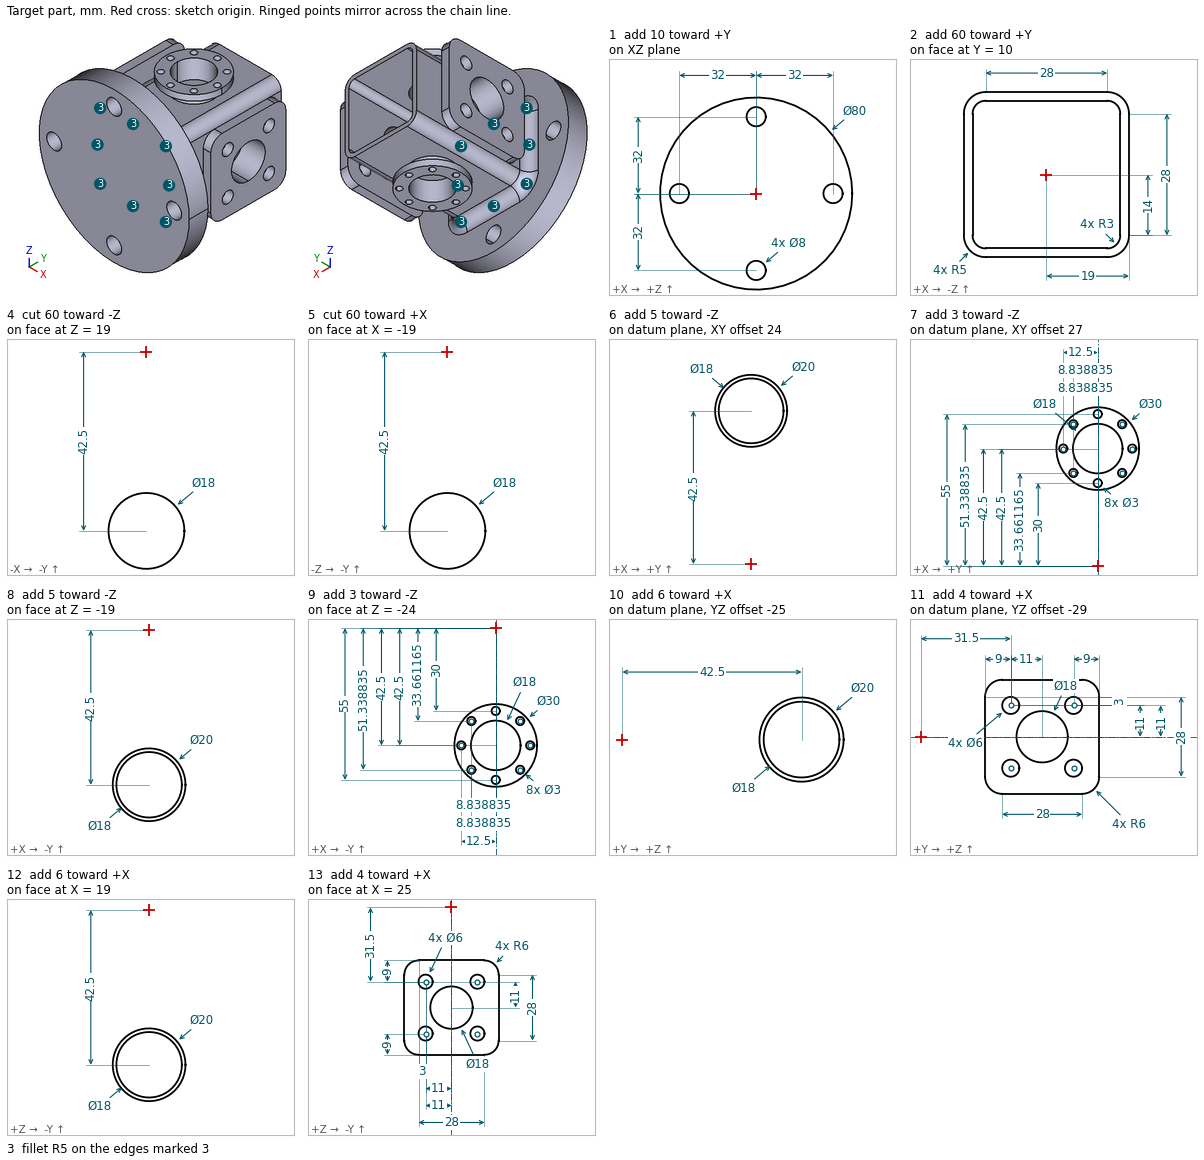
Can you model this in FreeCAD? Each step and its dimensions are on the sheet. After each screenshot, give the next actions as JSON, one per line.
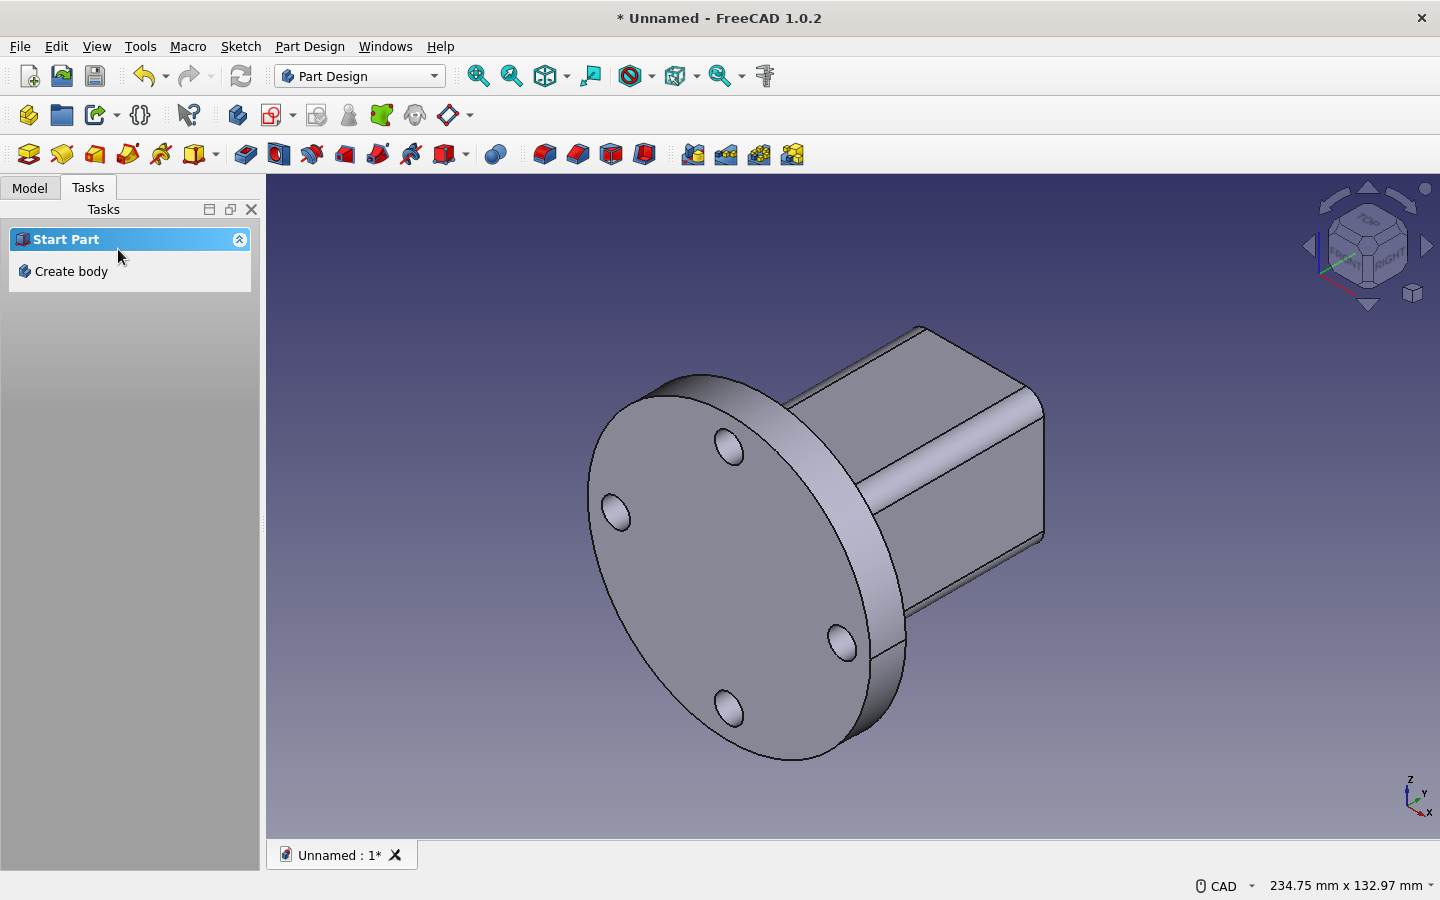
{"action": "key", "text": "2"}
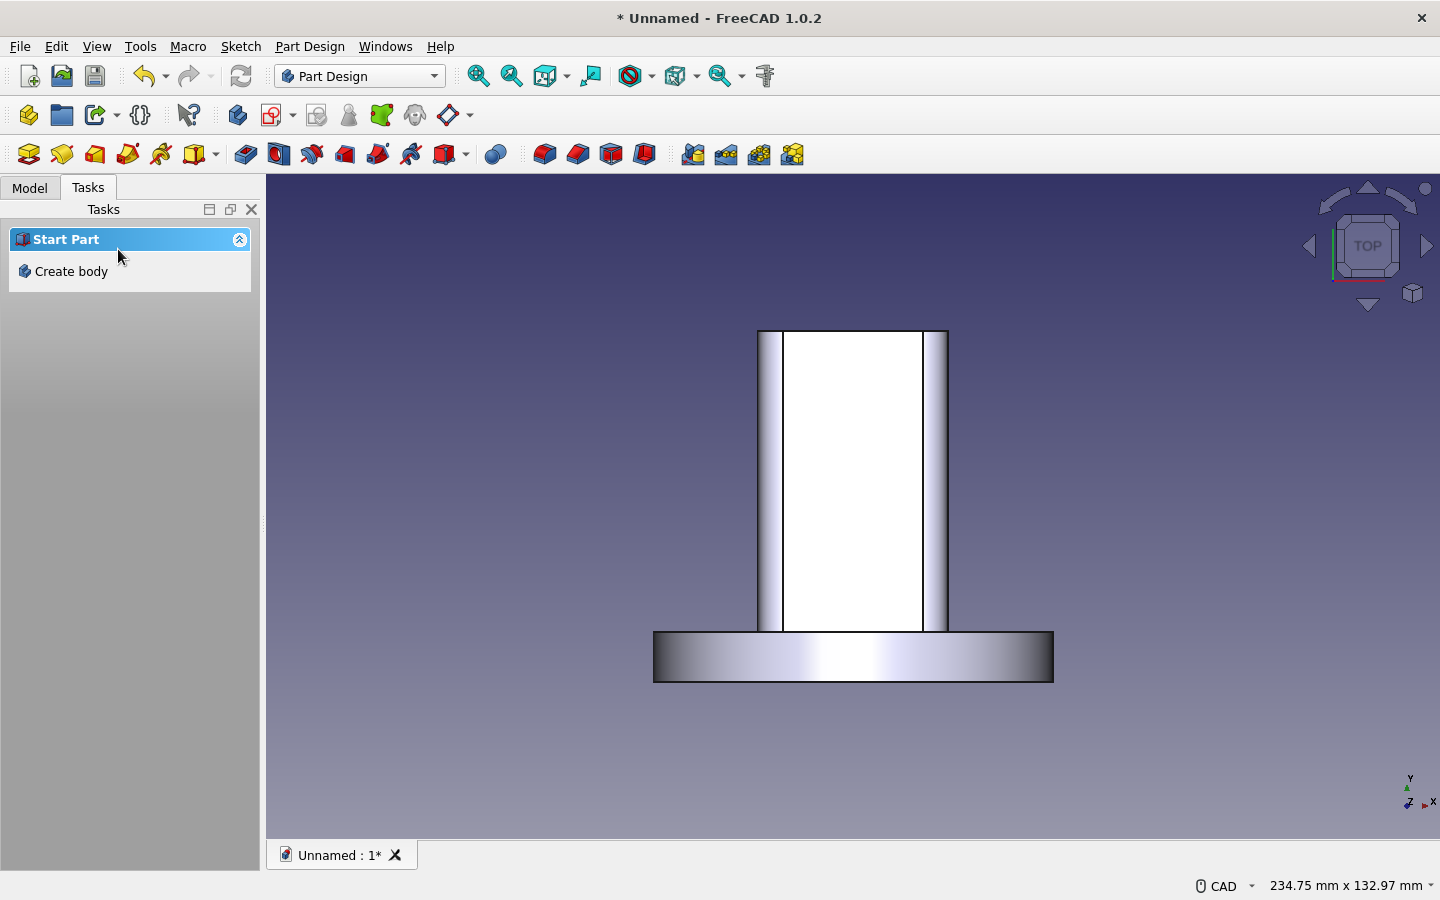
{"action": "key", "text": "1"}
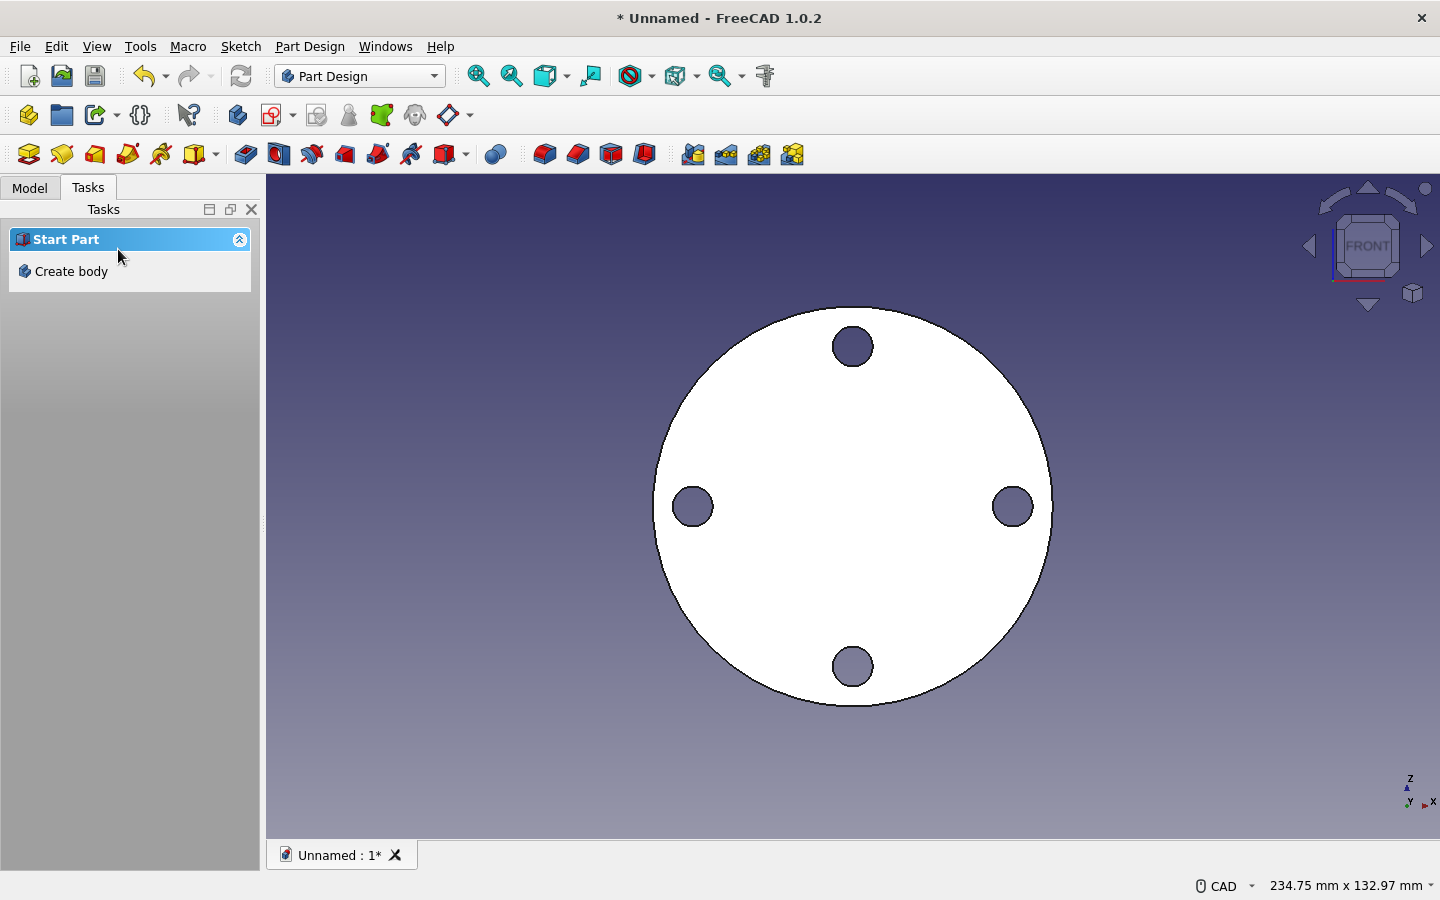
{"action": "key", "text": "3"}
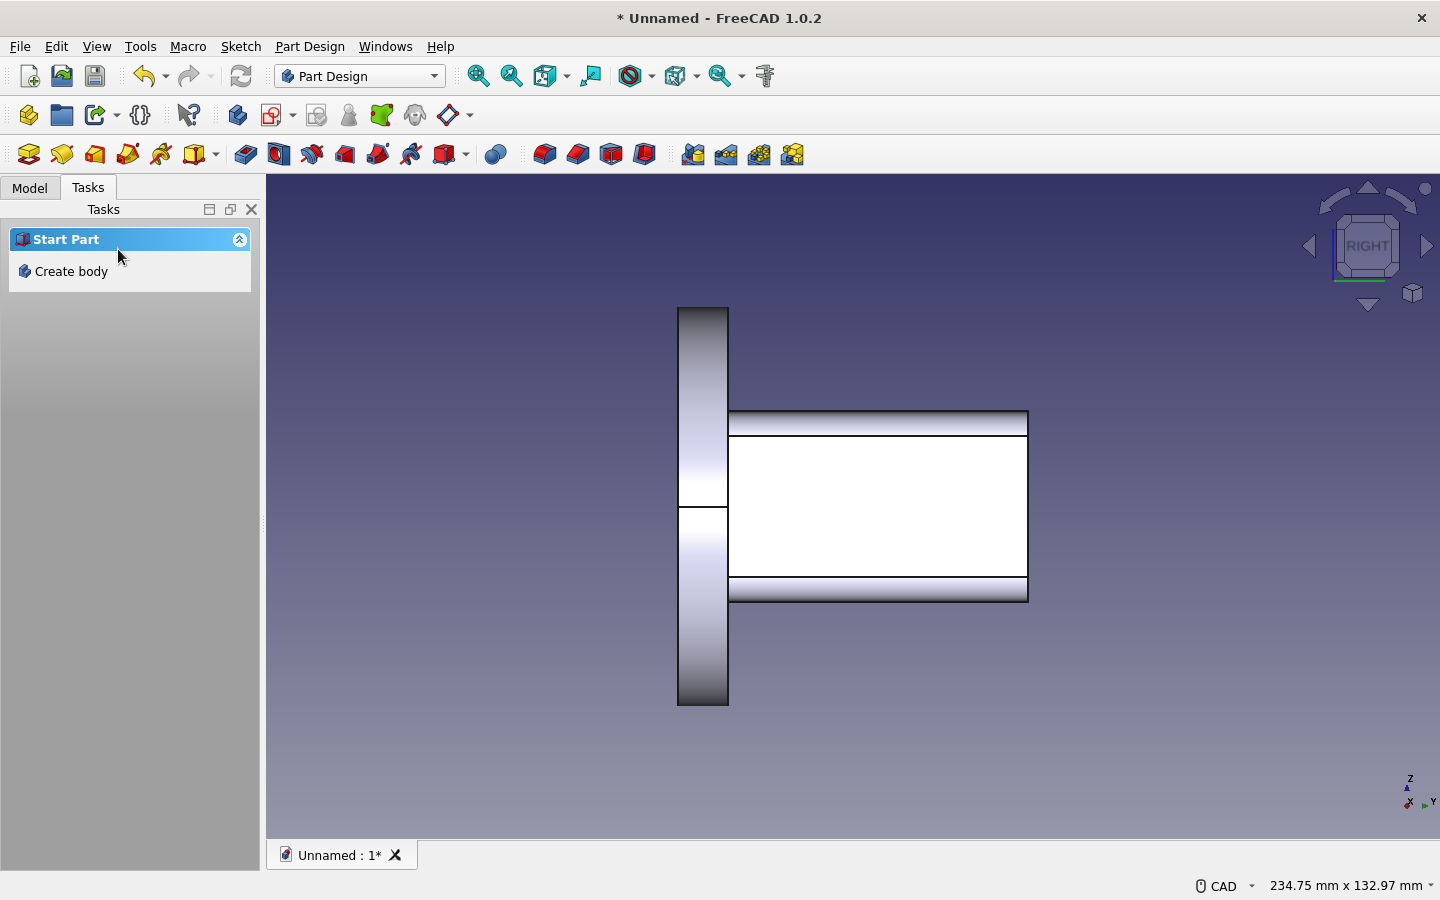
{"action": "key", "text": "5"}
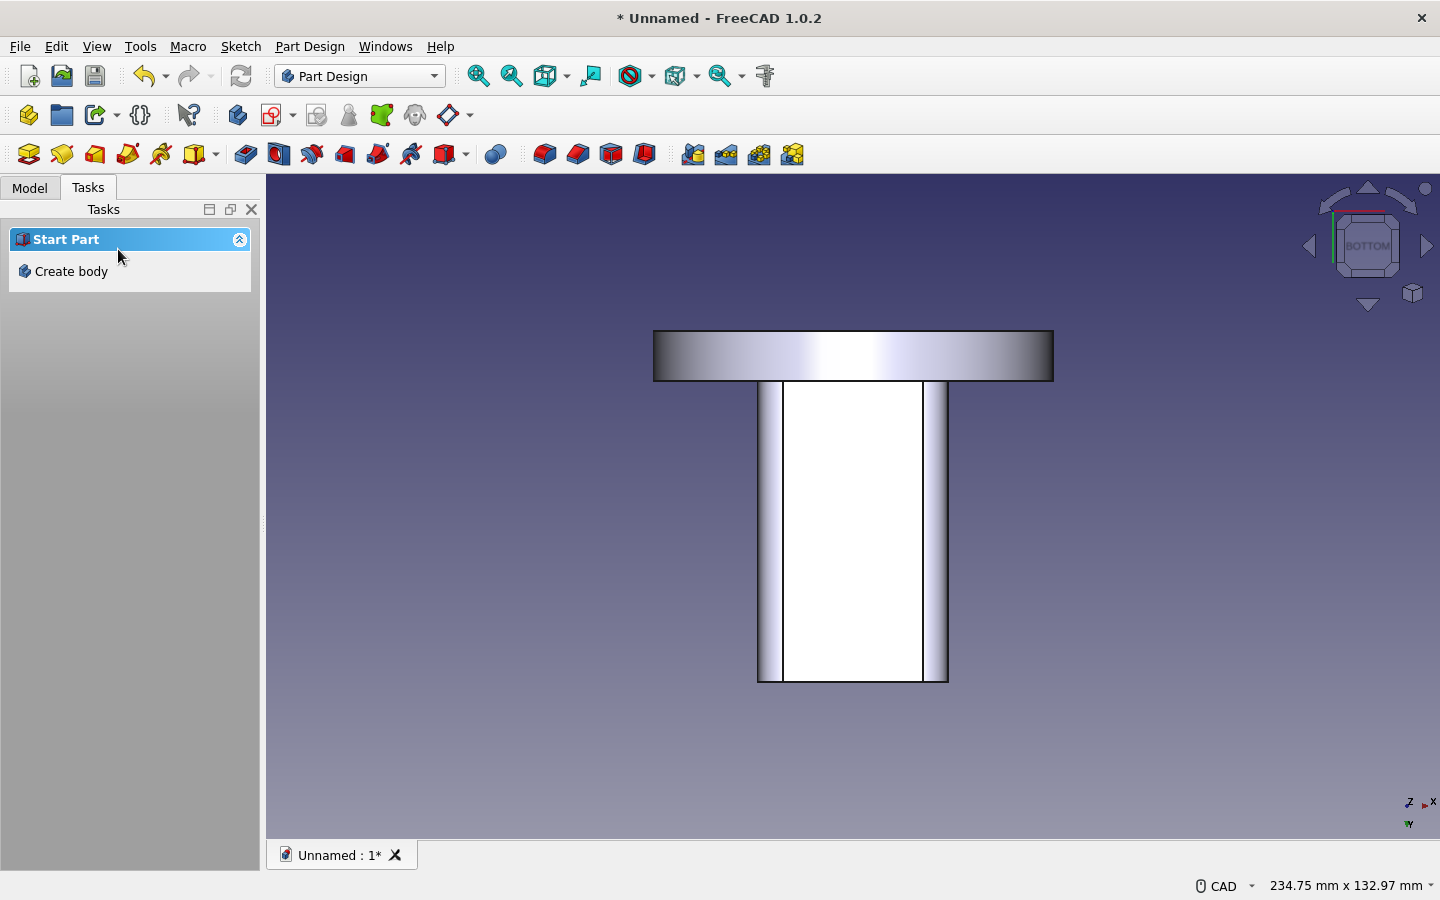
{"action": "key", "text": "4"}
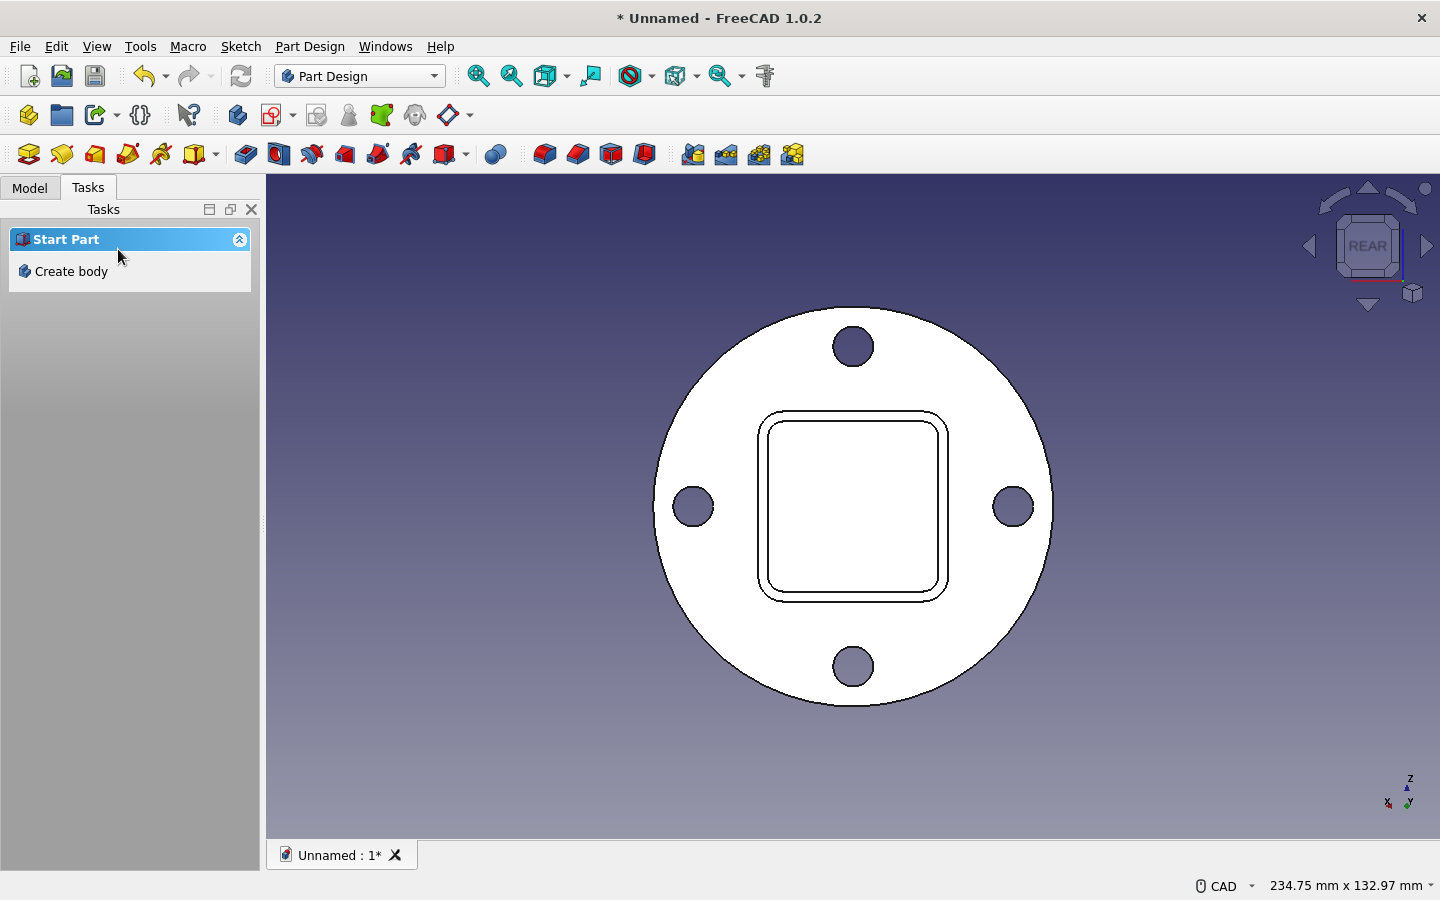
{"action": "key", "text": "6"}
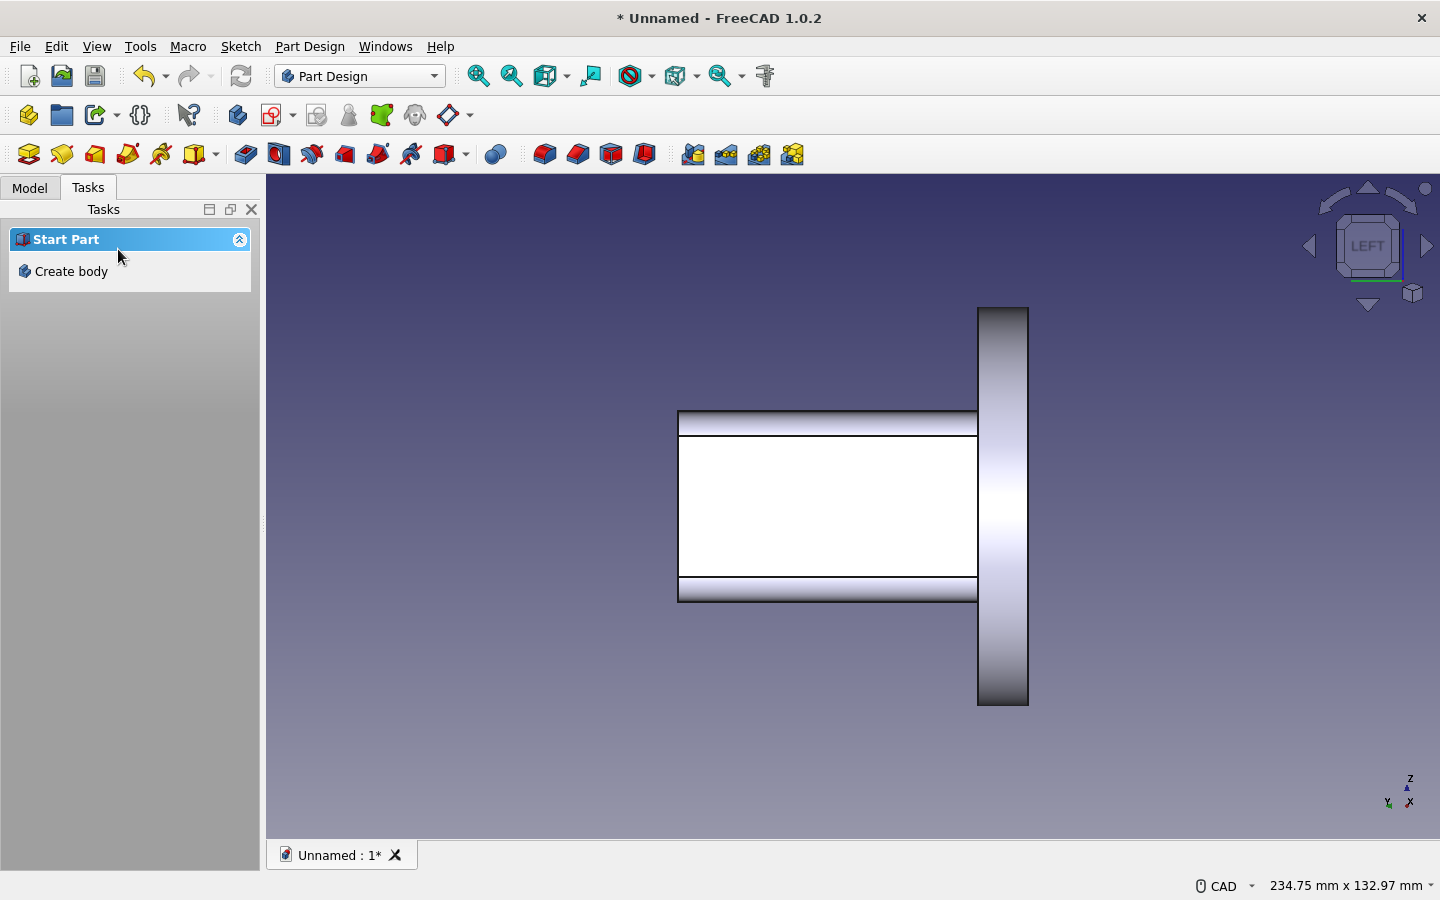
{"action": "key", "text": "v 3"}